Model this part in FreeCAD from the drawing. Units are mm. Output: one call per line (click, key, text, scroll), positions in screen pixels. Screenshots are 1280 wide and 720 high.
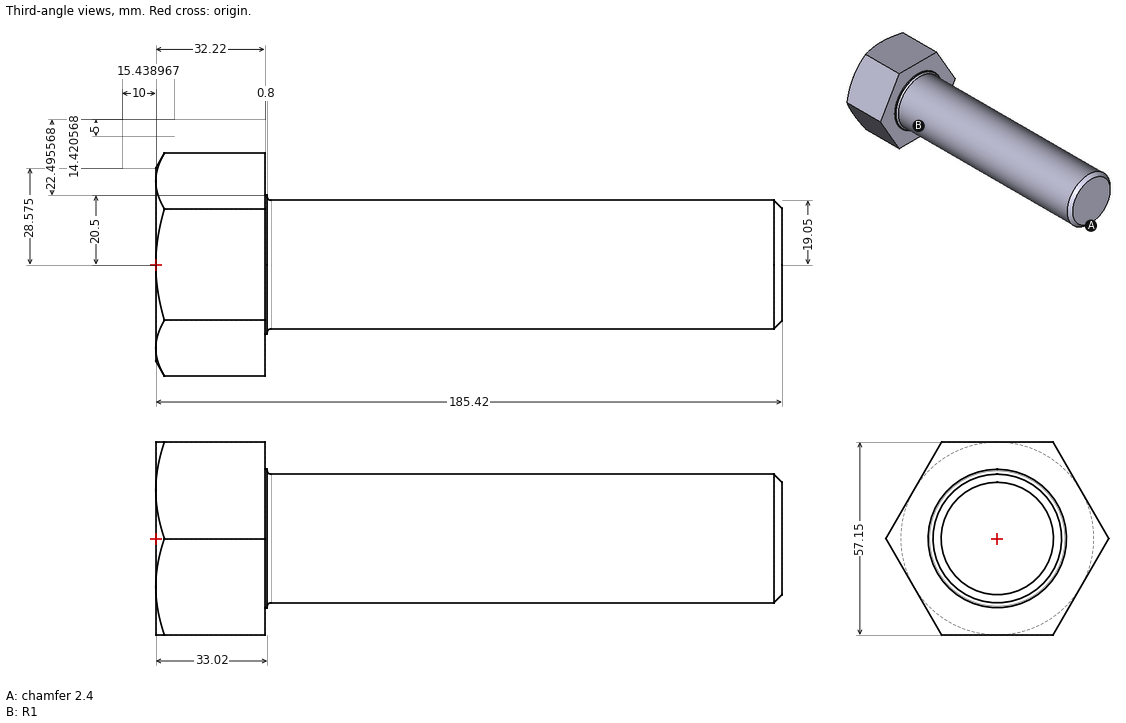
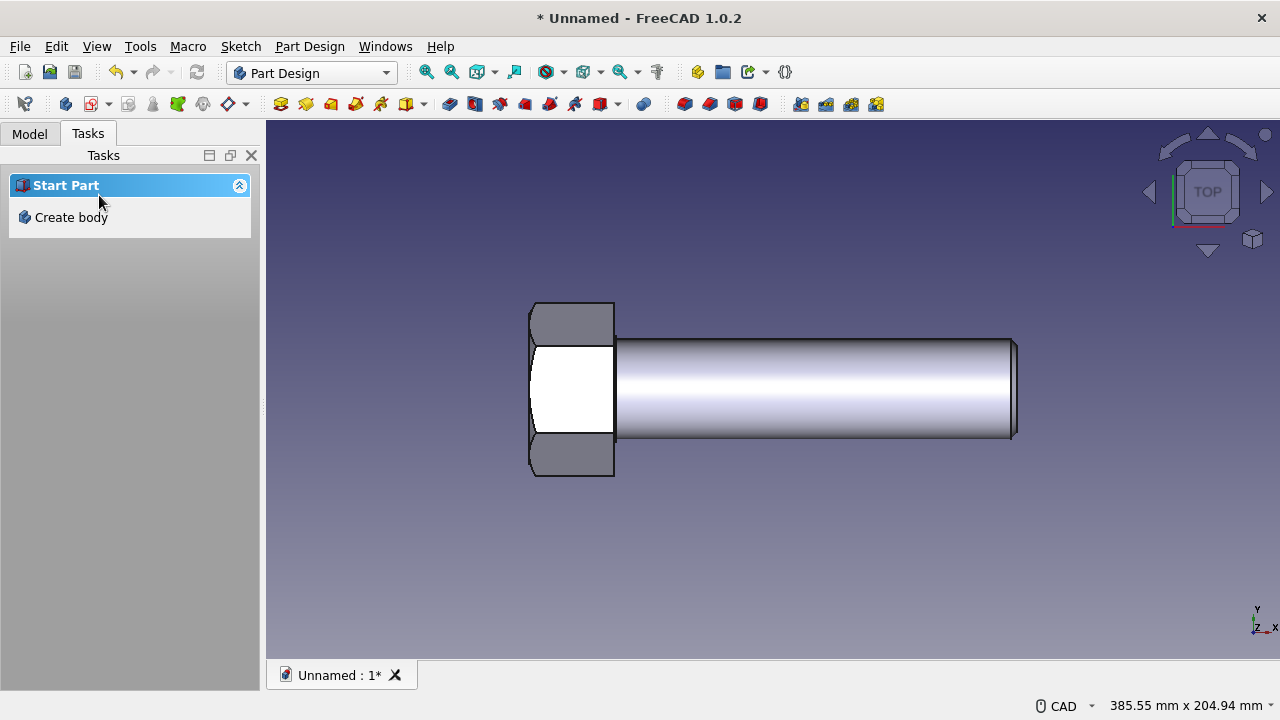
key(1)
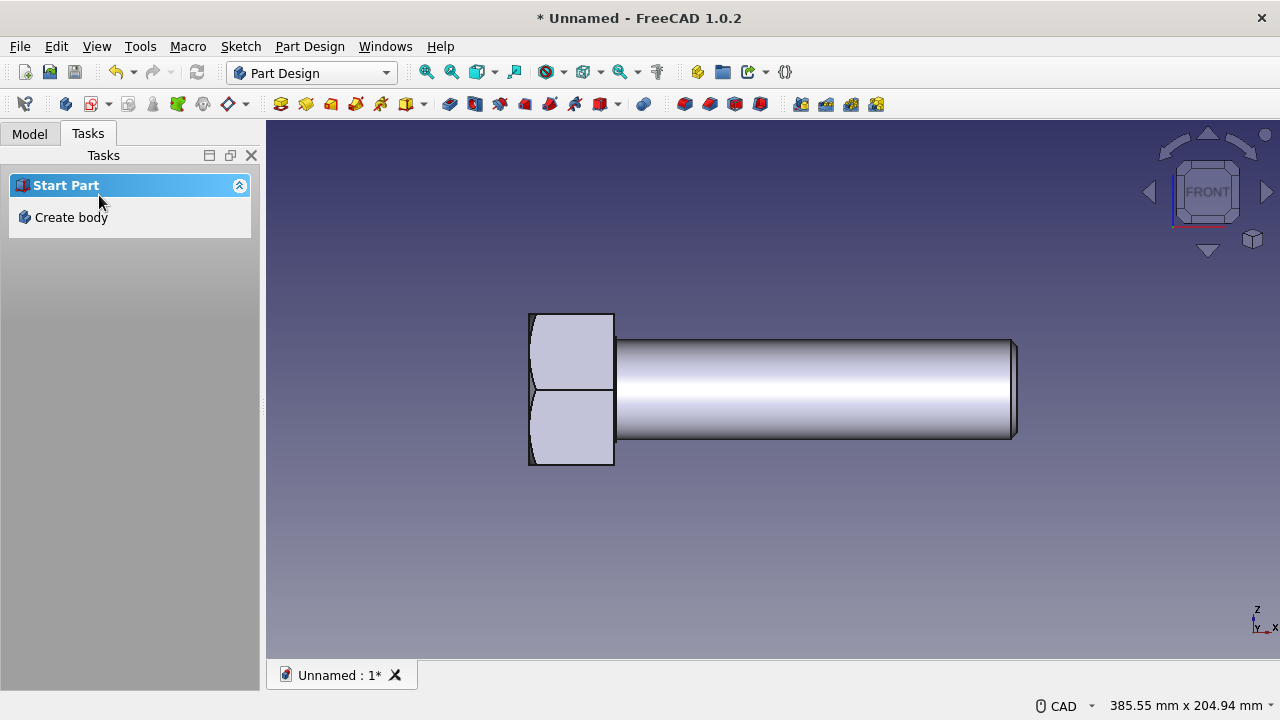
key(3)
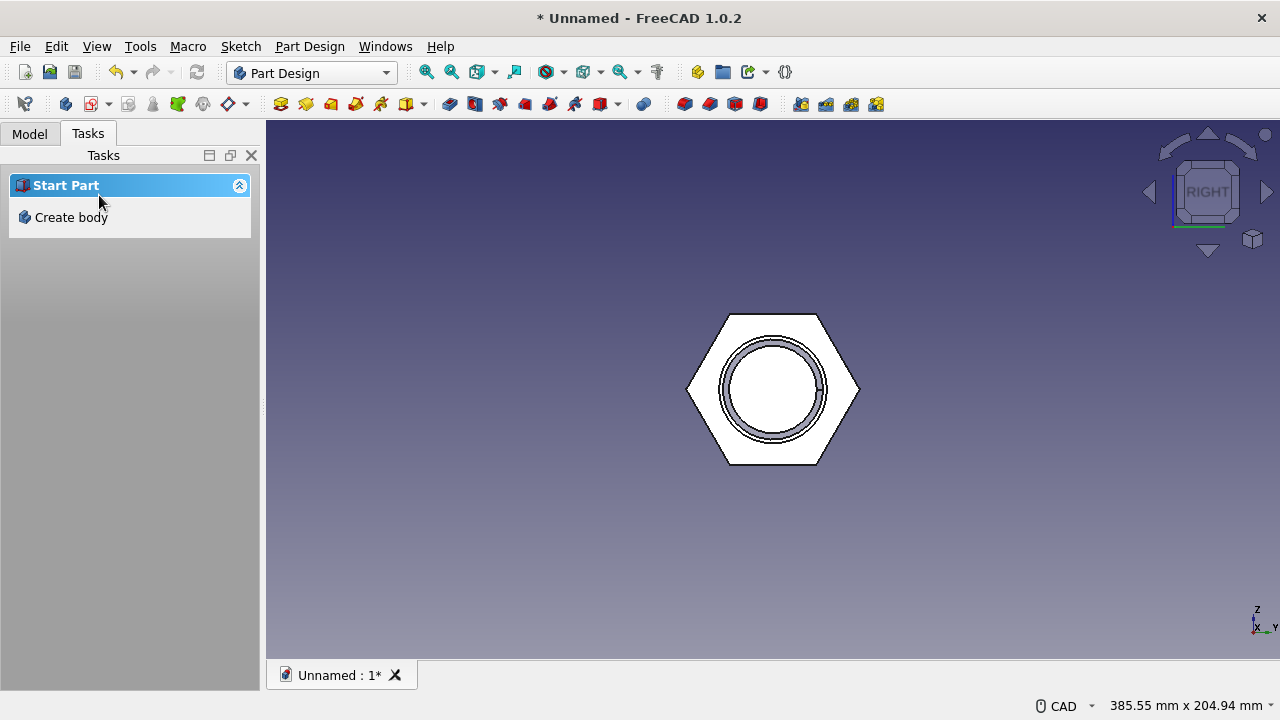
key(v)
key(f)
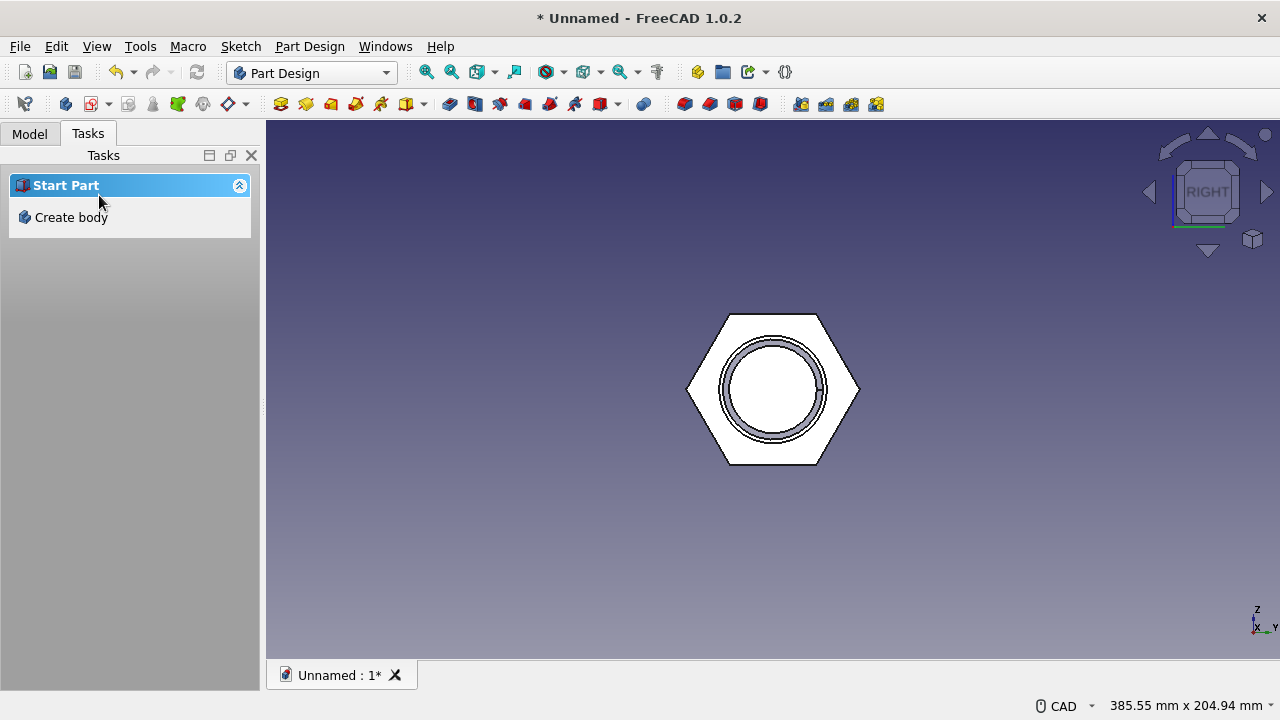
key(5)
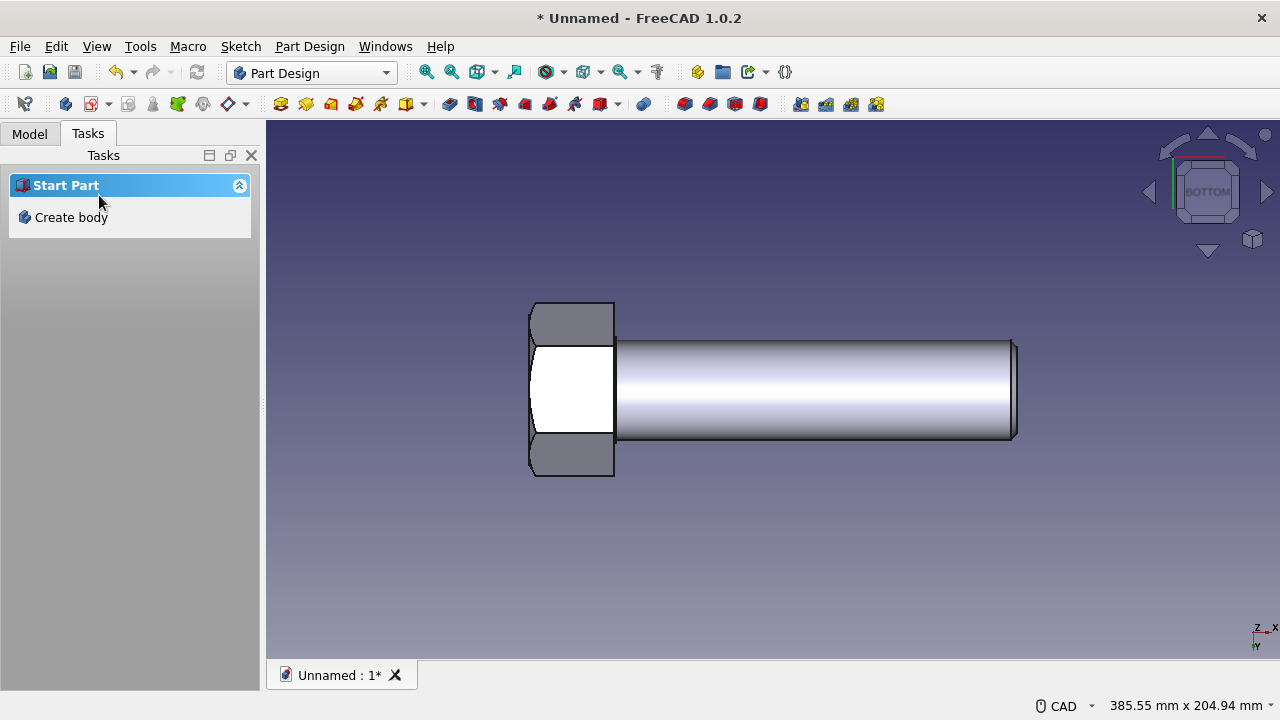
key(4)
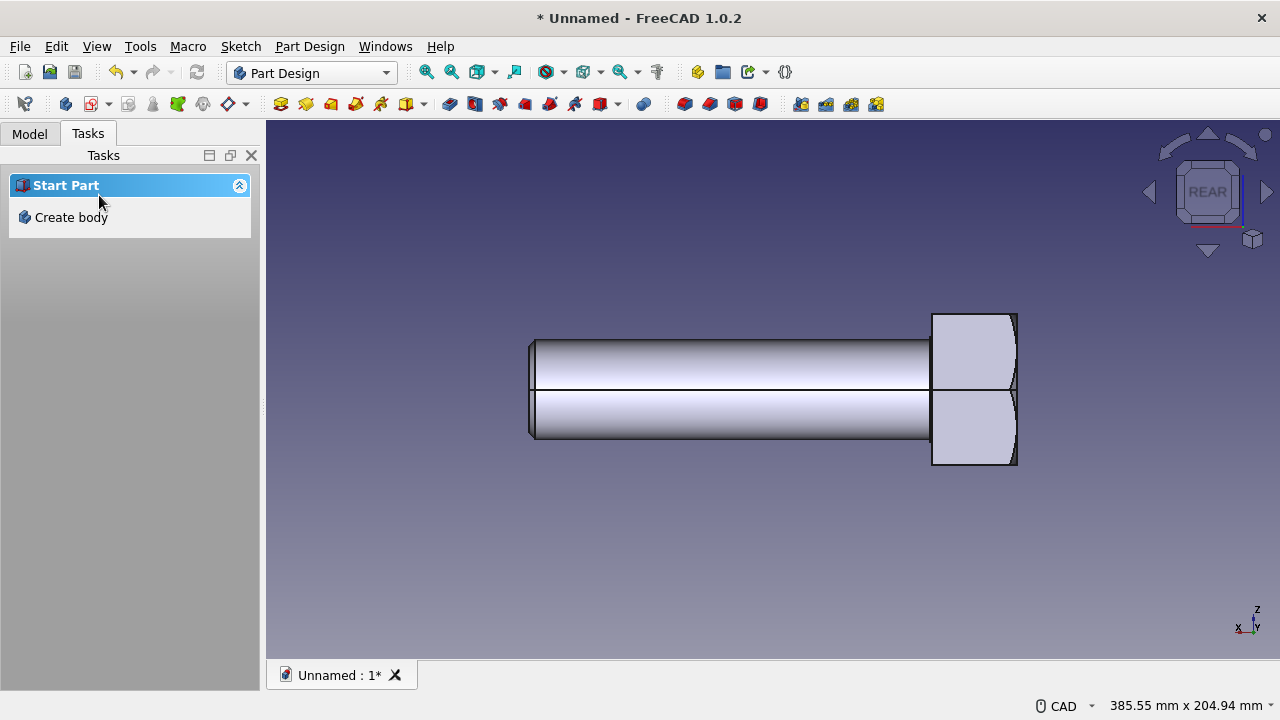
key(6)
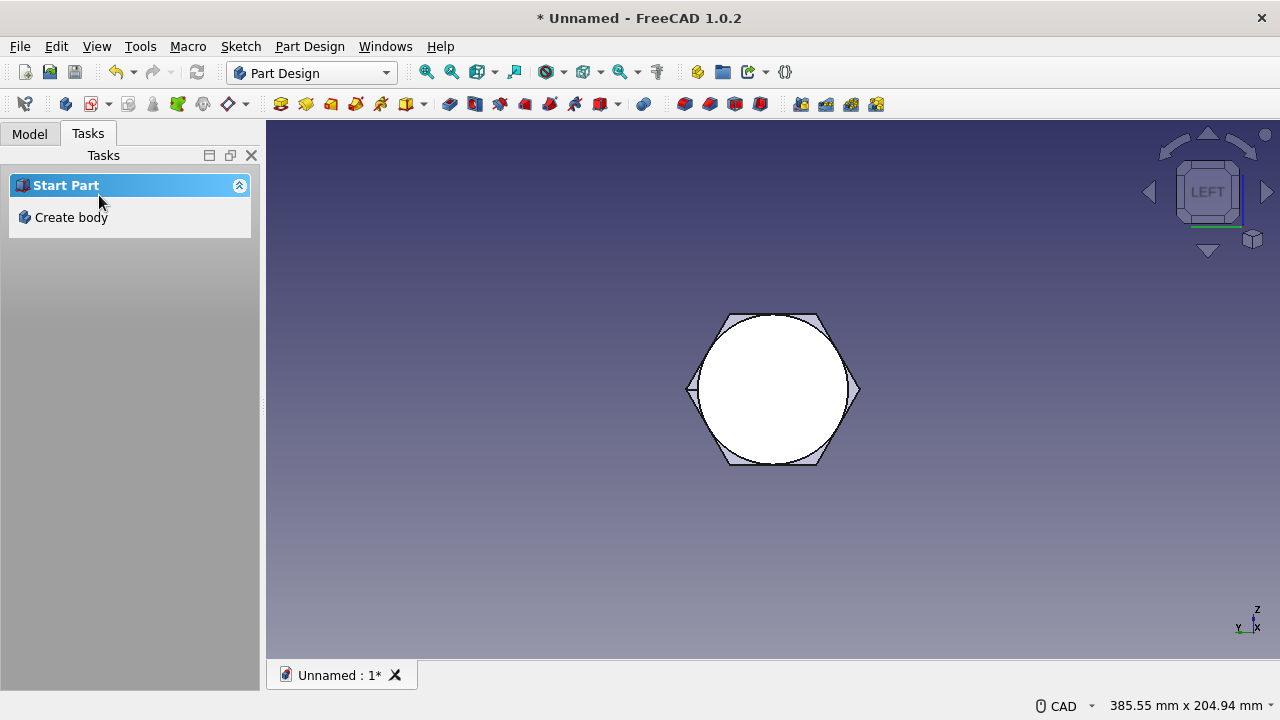
key(v)
key(f)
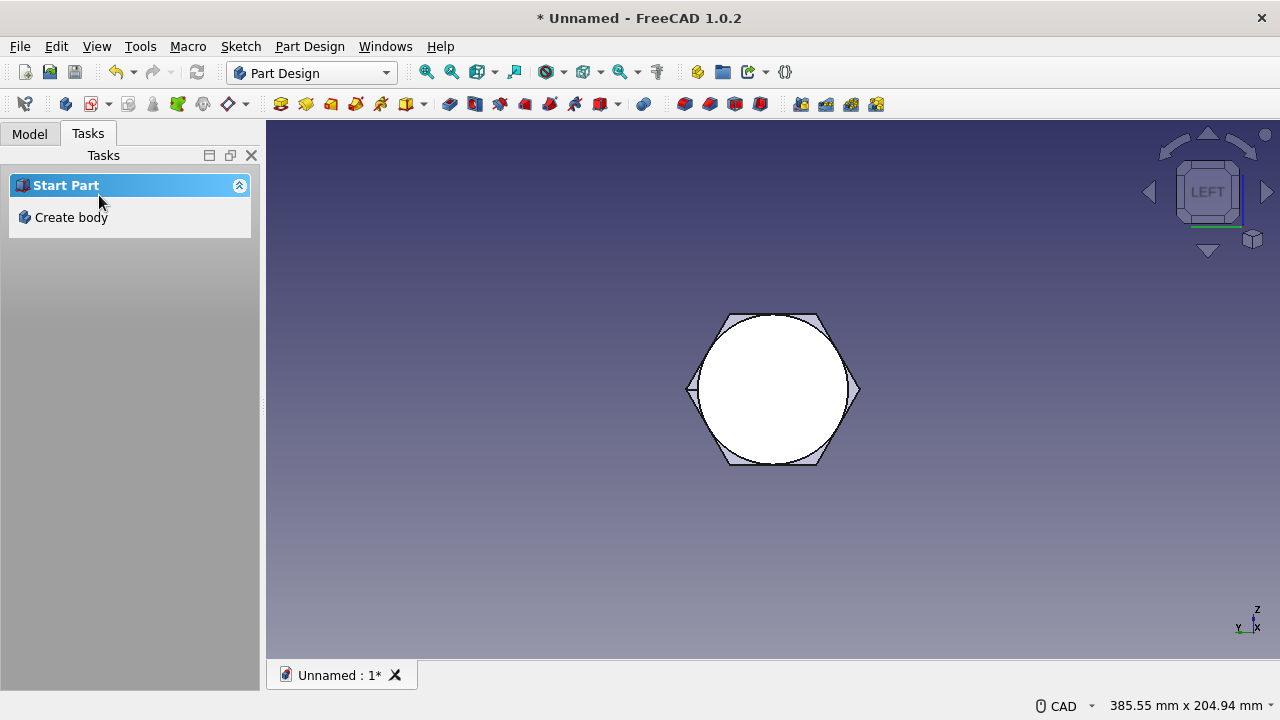
key(v)
key(3)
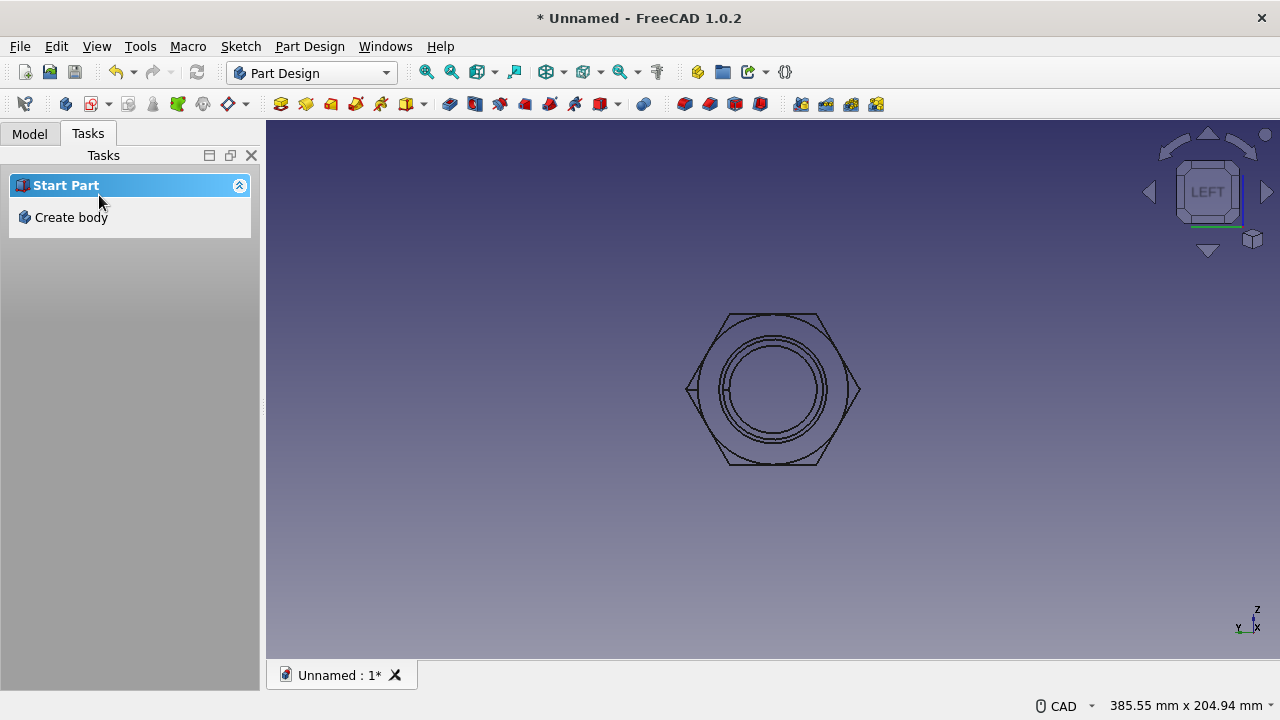
key(0)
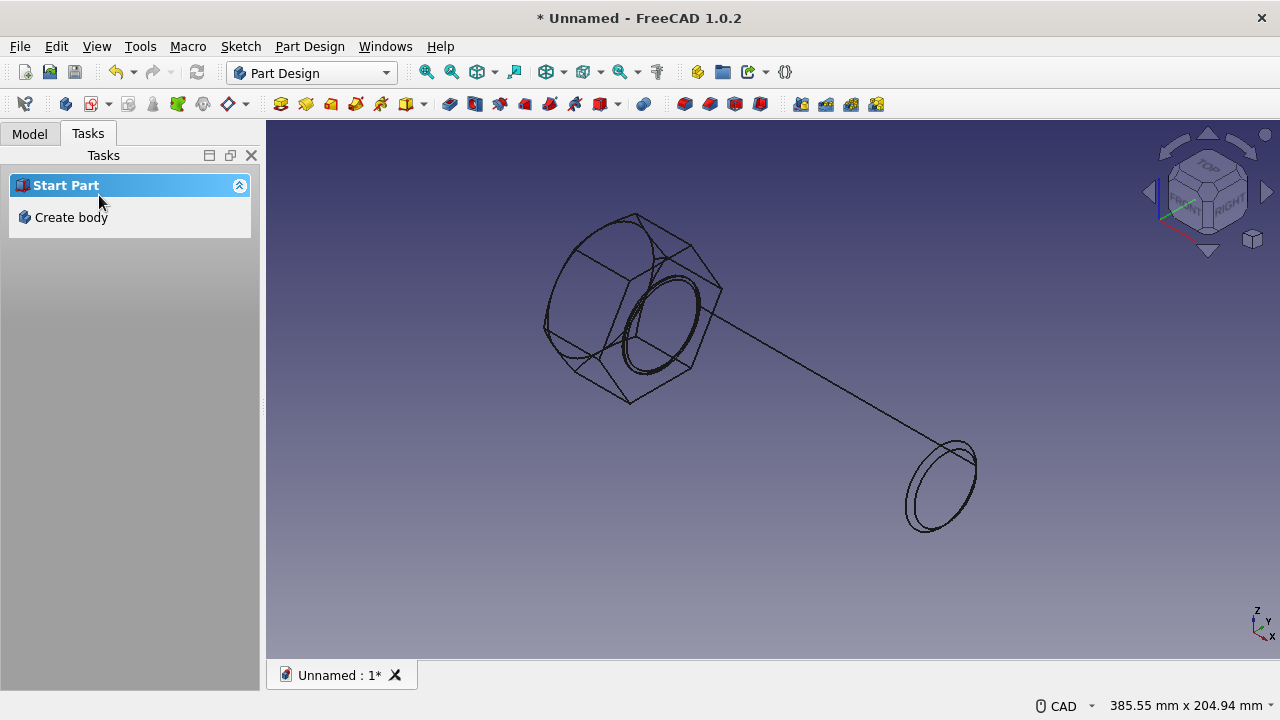
click(673, 357)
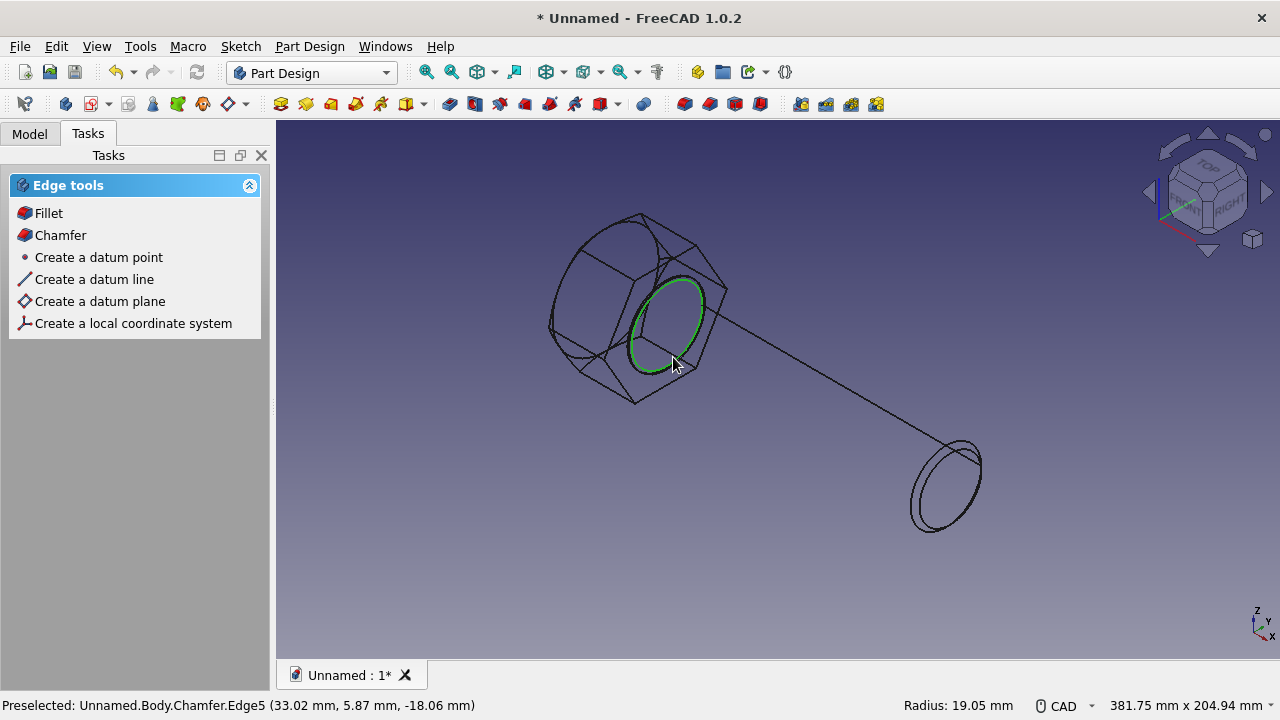
key(v)
key(1)